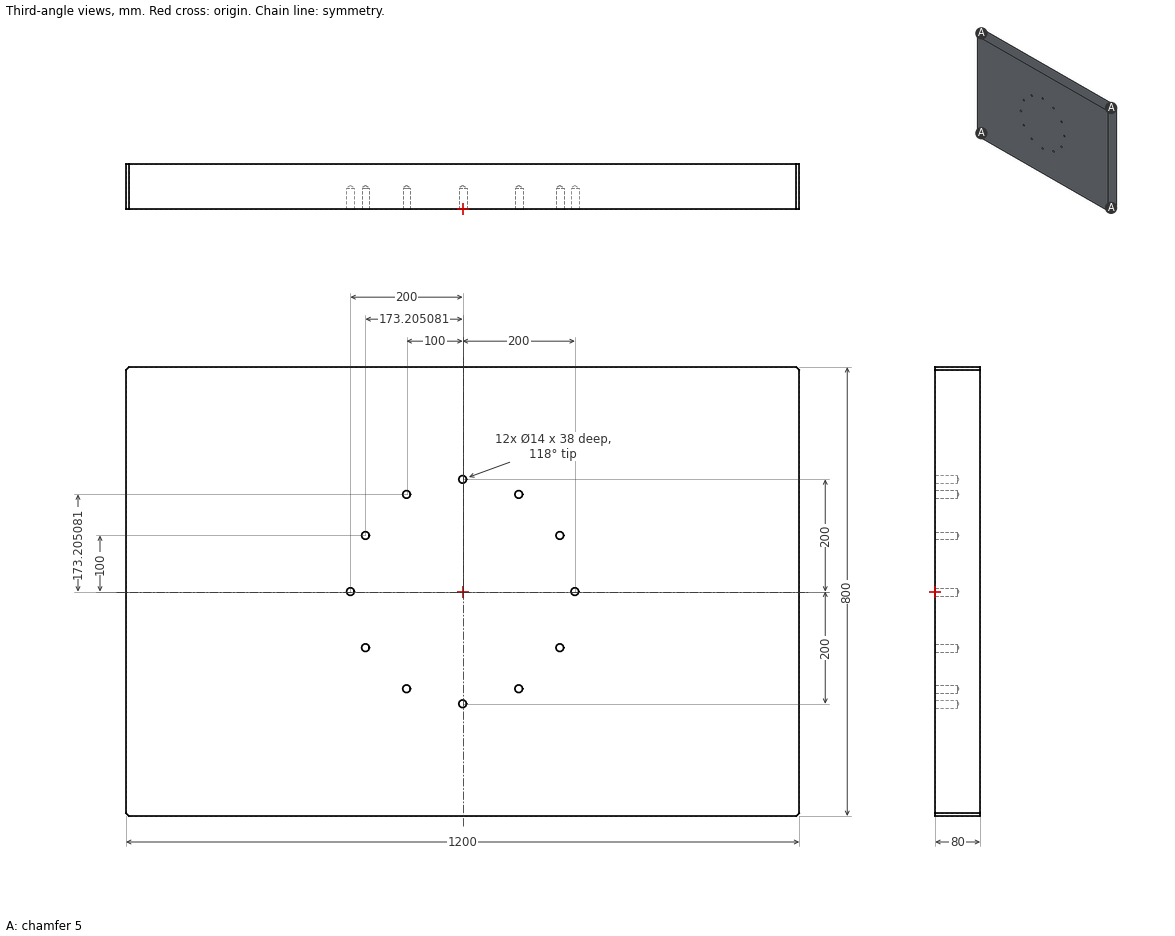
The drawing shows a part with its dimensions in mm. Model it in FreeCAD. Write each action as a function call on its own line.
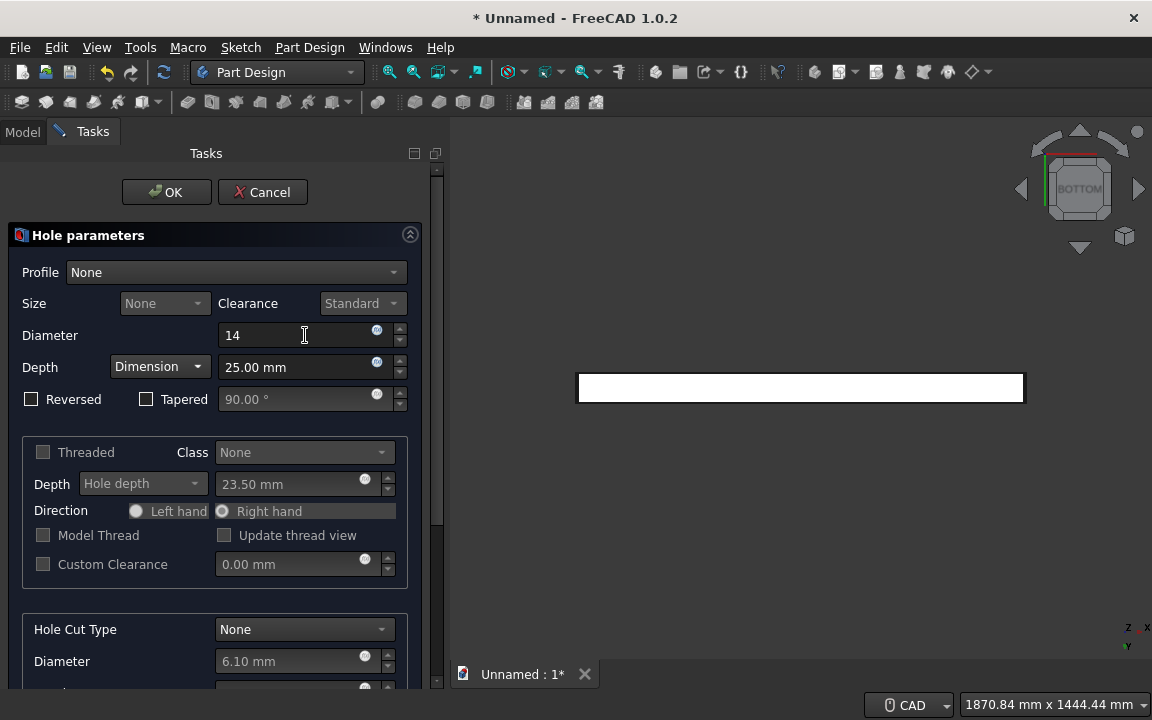
triple_click(305, 367)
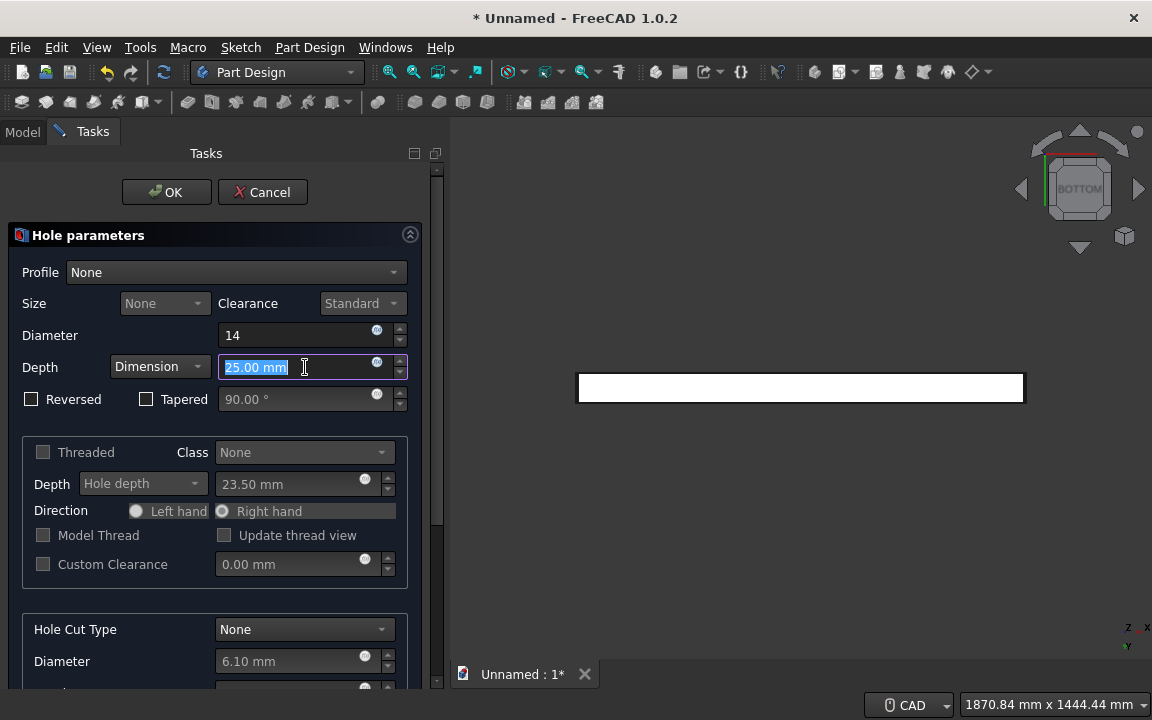
text(38)
key(Tab)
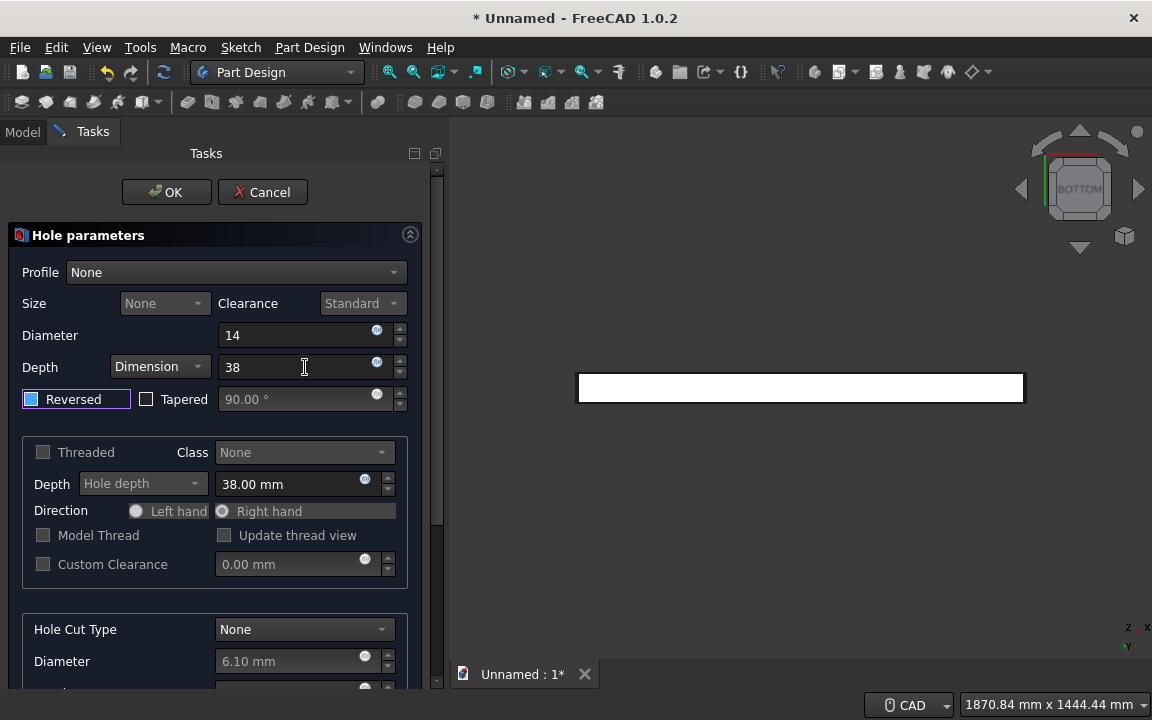
click(167, 192)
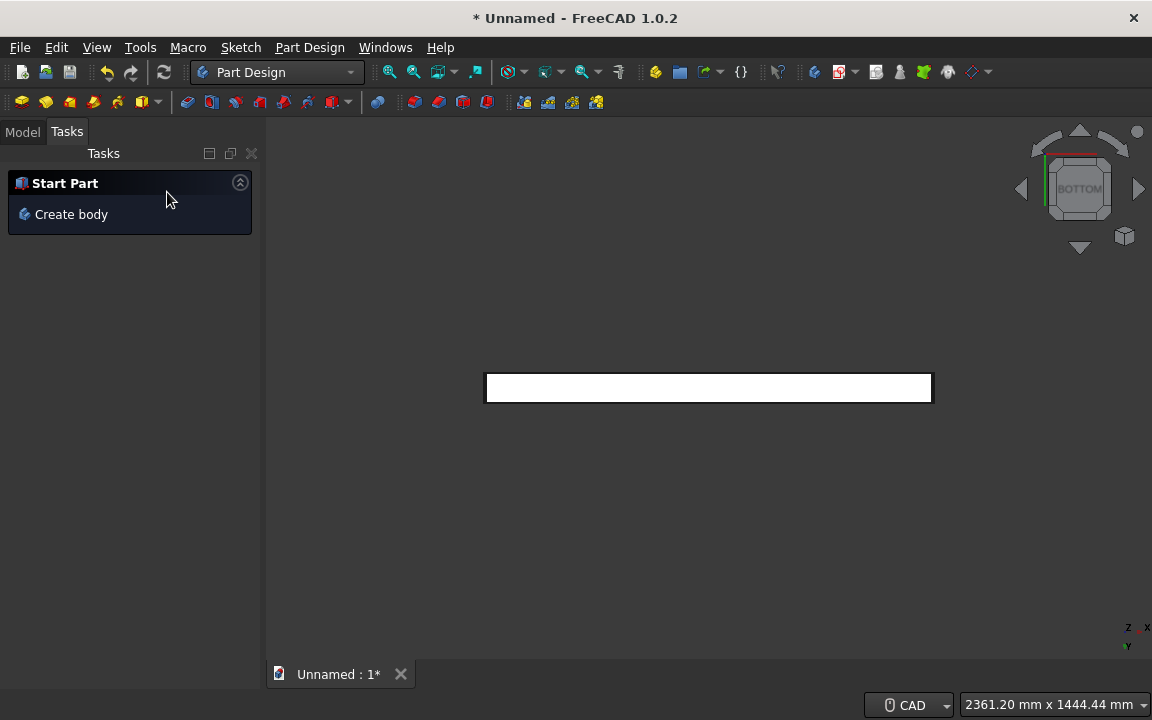
key(0)